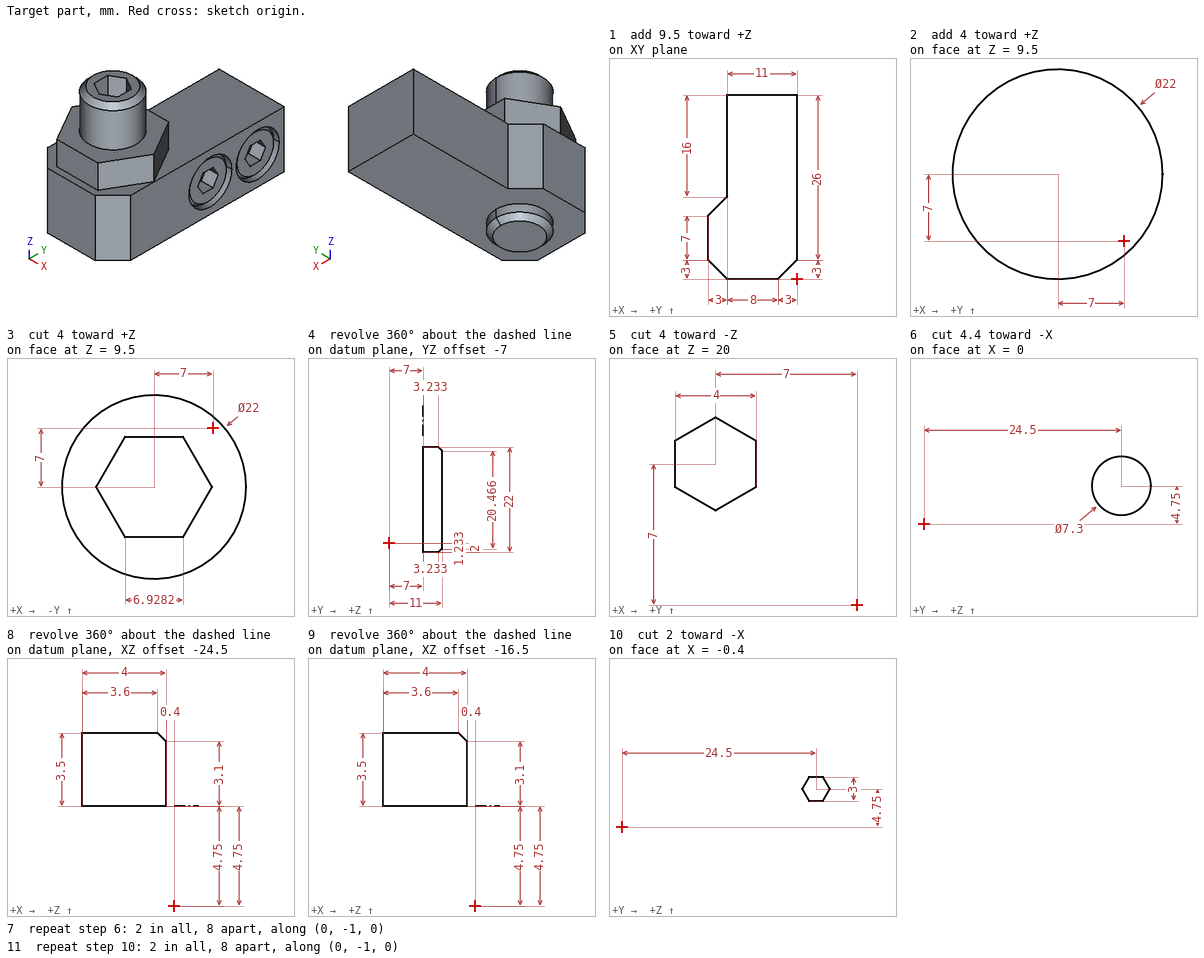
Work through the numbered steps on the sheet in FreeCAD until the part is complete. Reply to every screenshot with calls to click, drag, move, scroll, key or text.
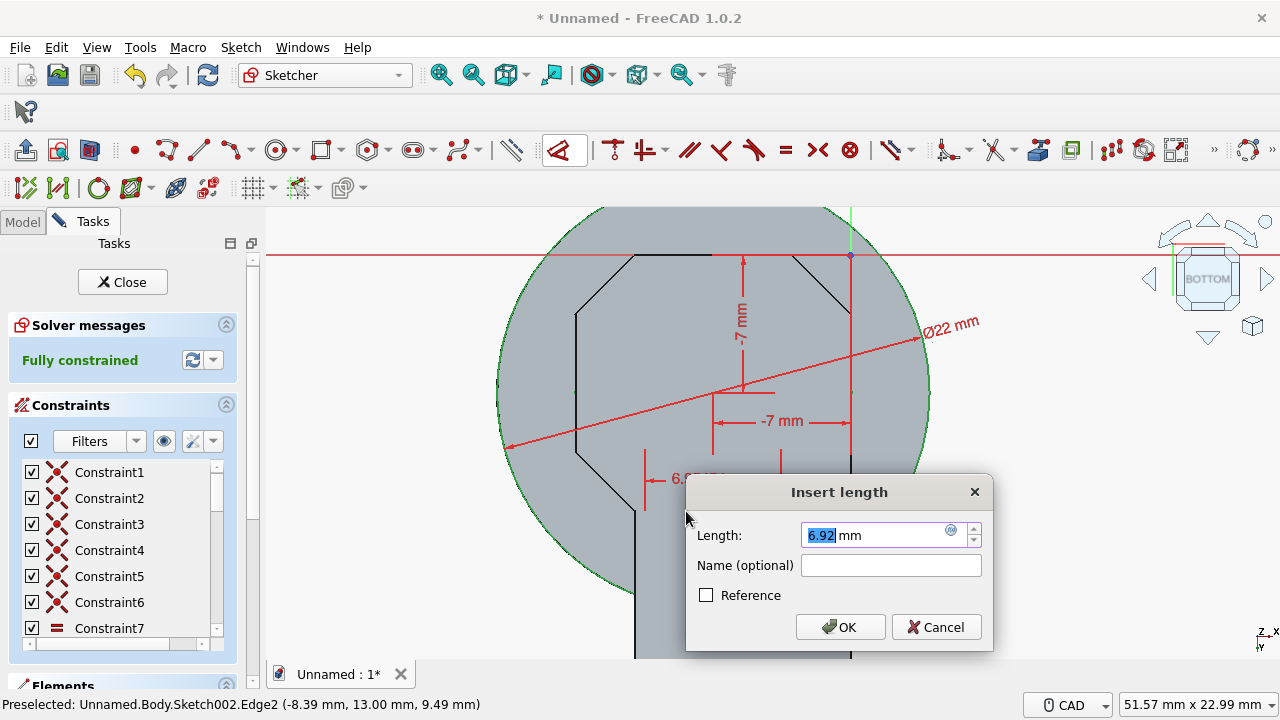
text(6.9282)
key(Return)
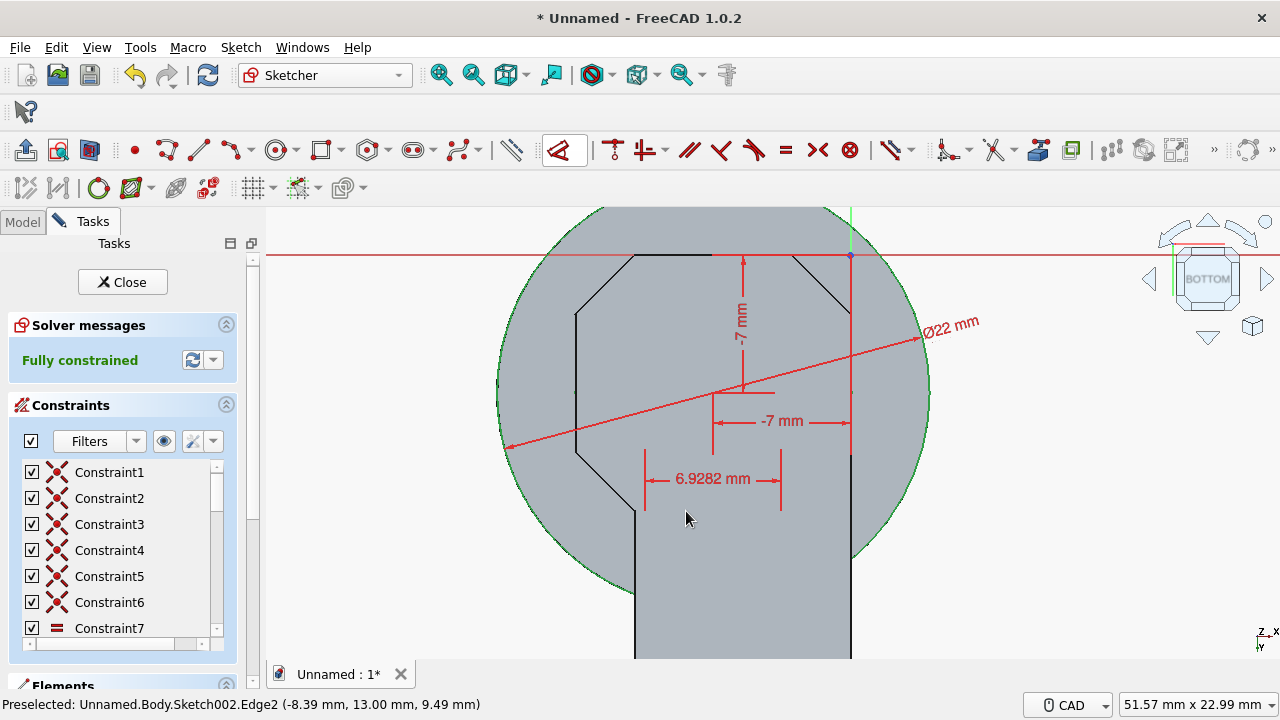
click(123, 282)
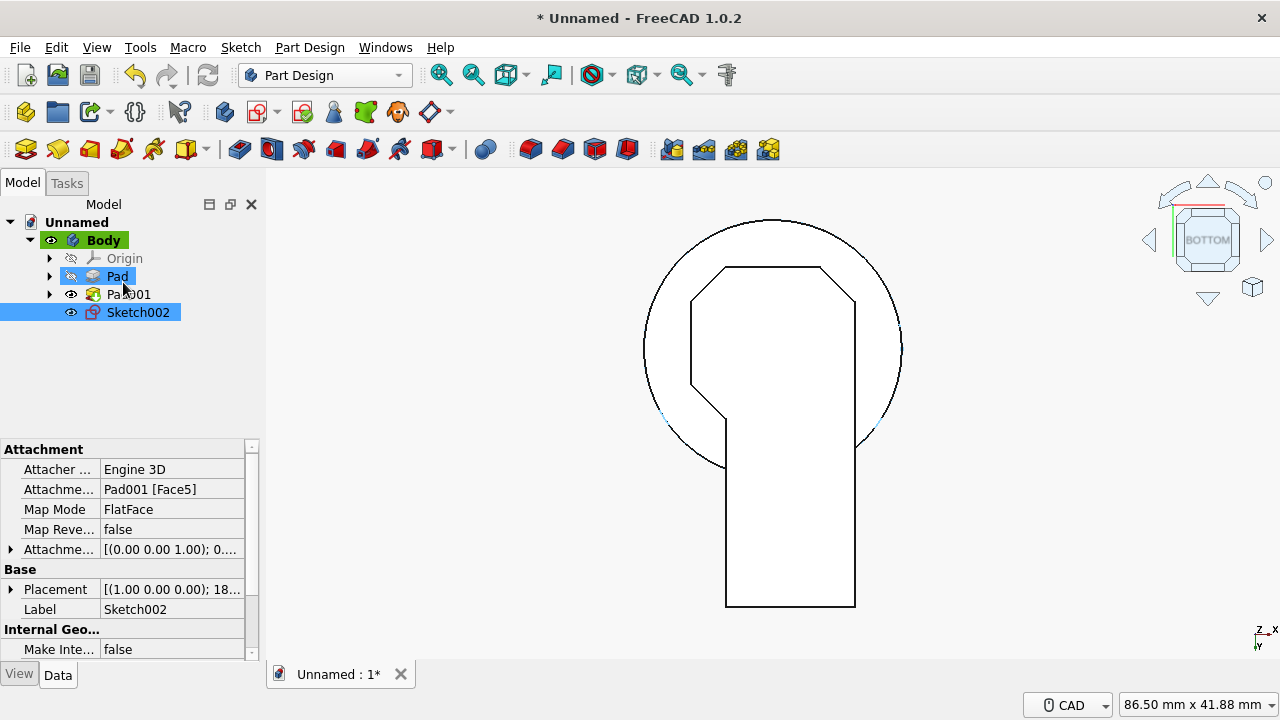
click(240, 150)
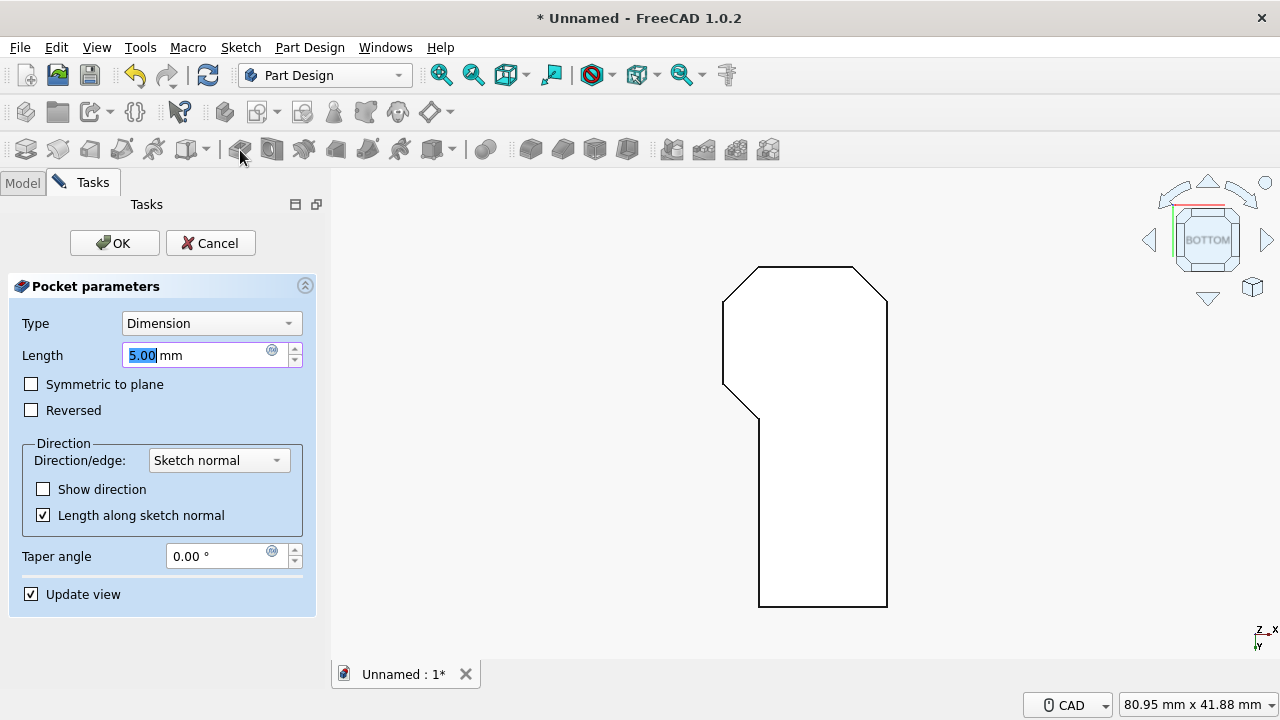
text(4)
key(Tab)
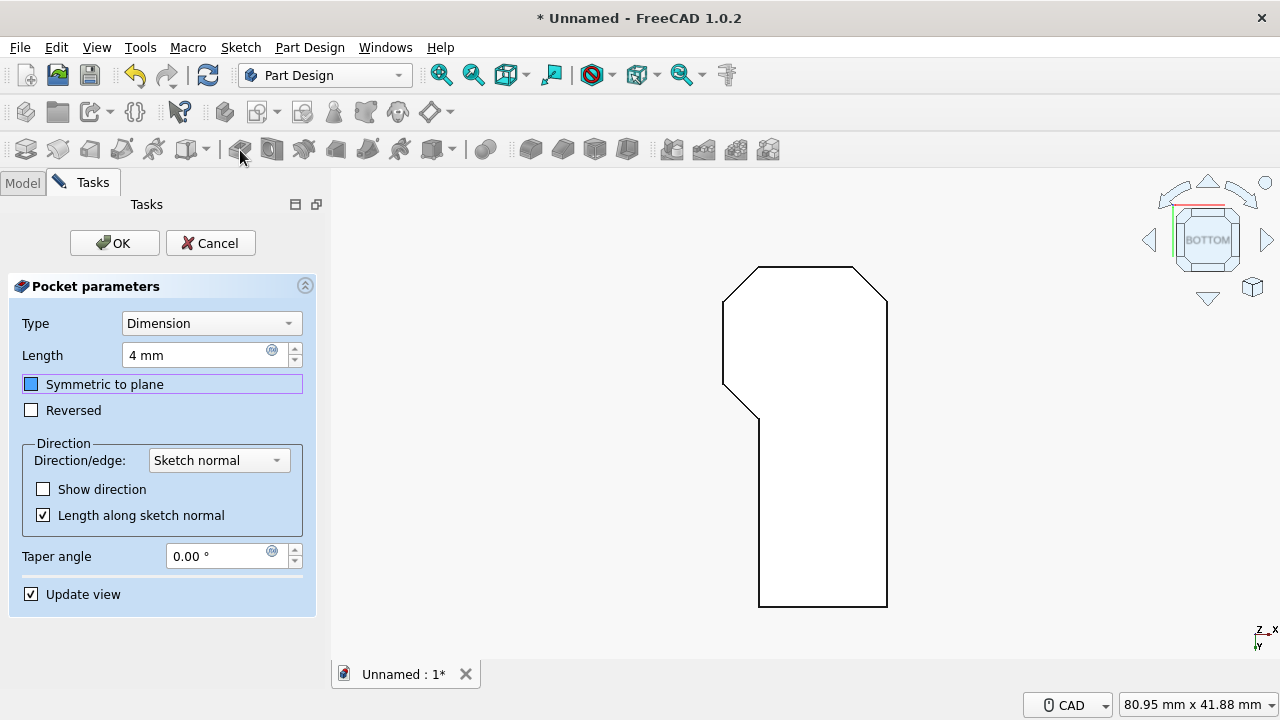
click(115, 243)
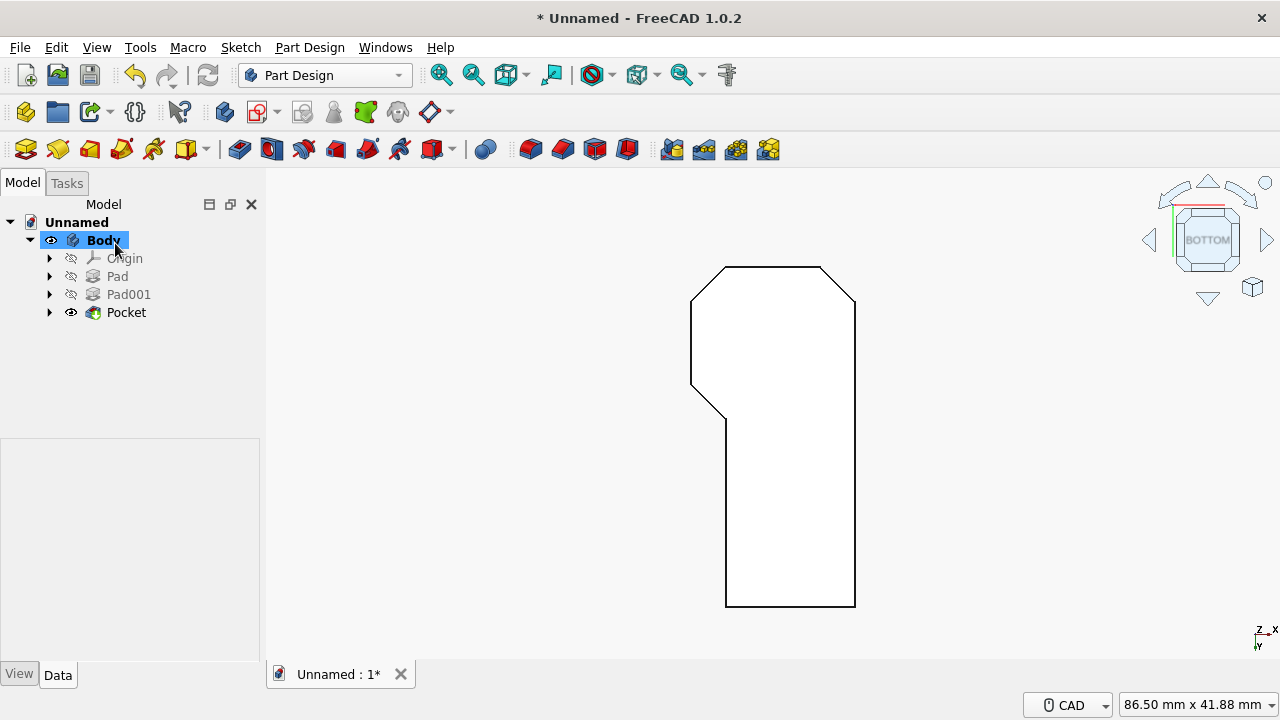
click(50, 258)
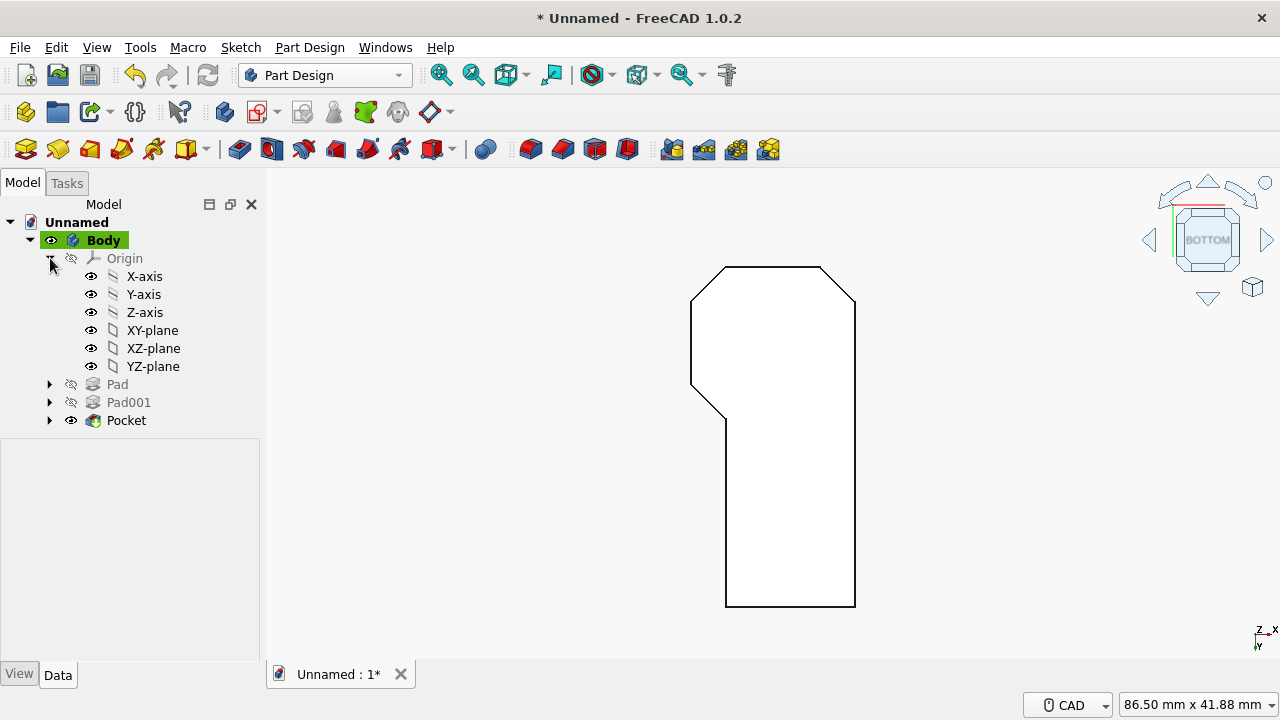
click(136, 366)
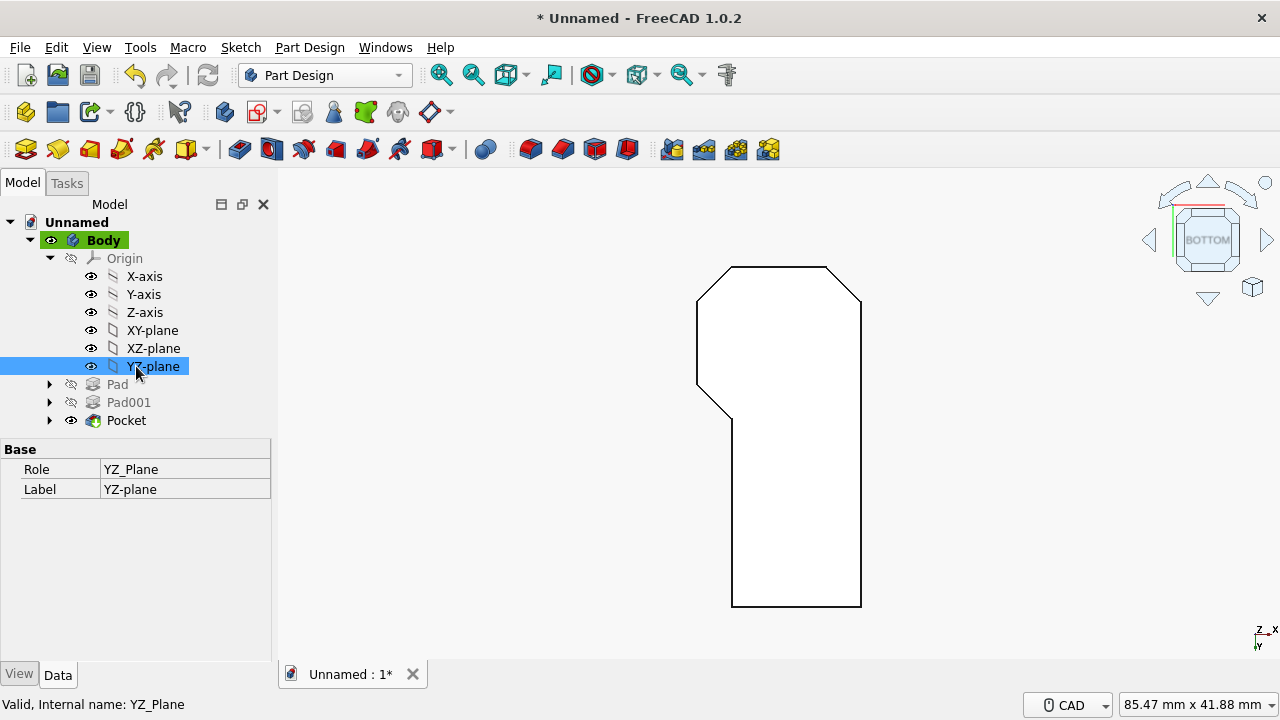
click(430, 112)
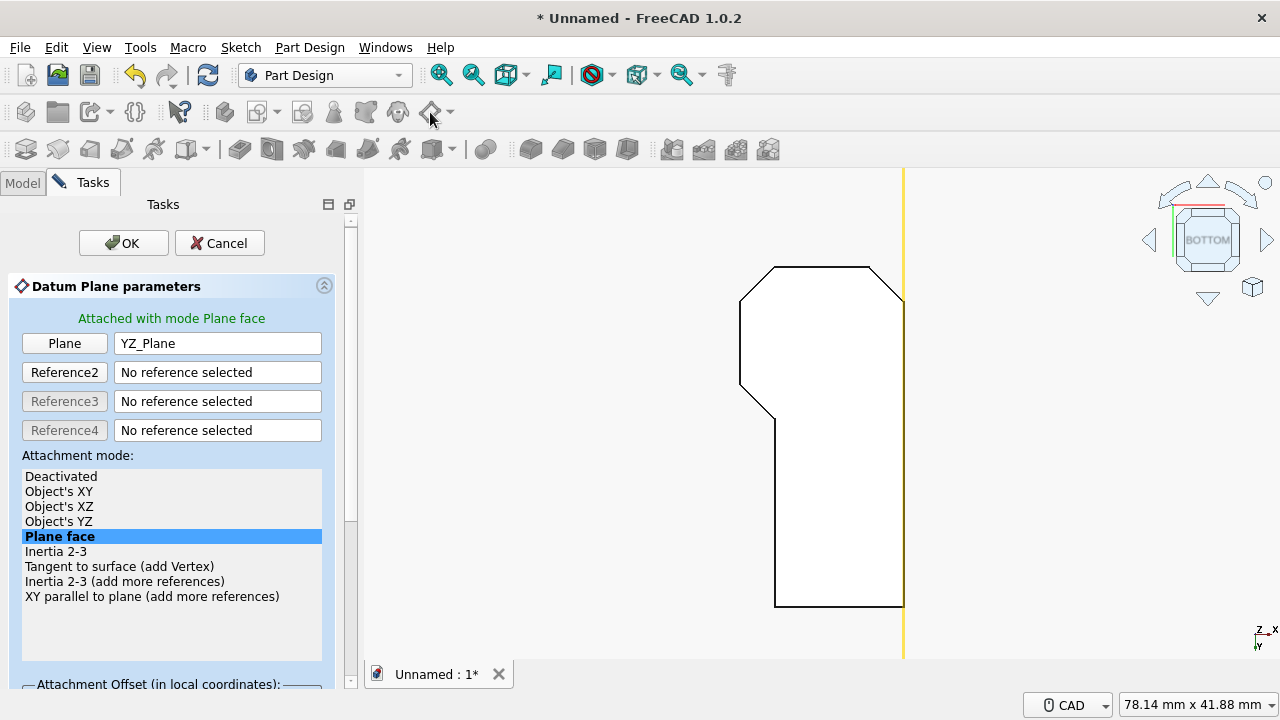
scroll(351, 451, down, 3)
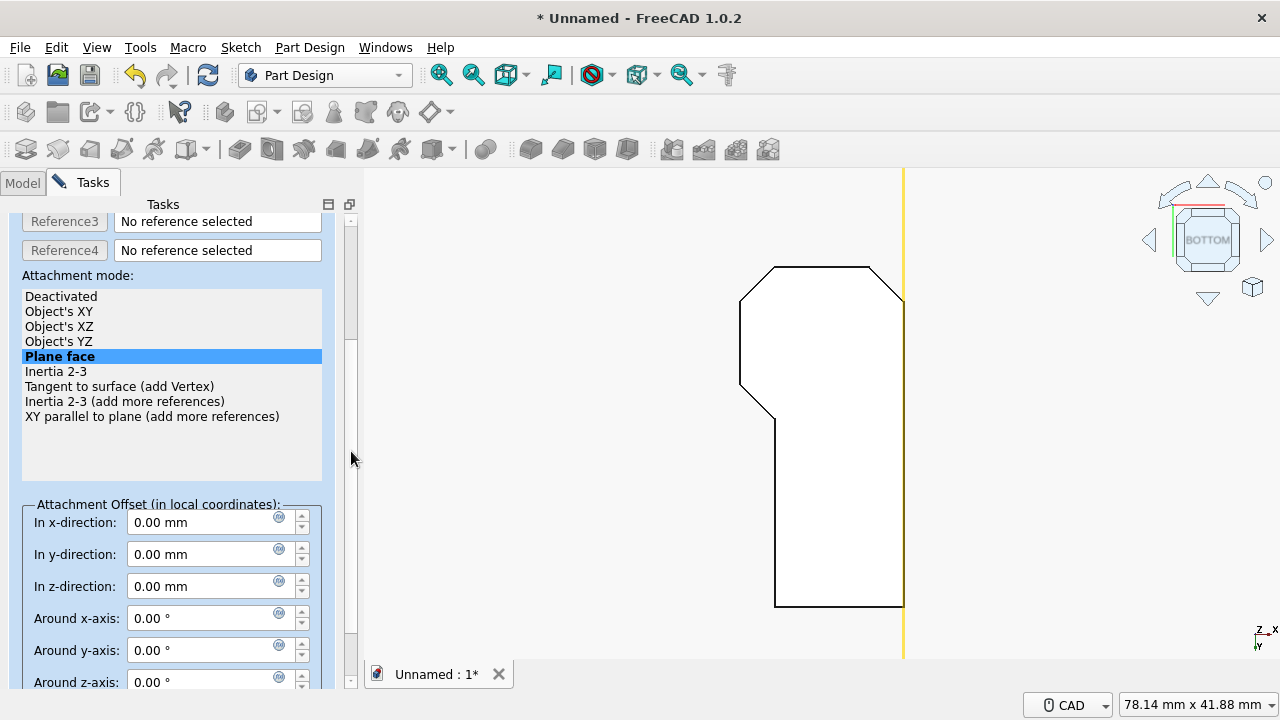
triple_click(210, 586)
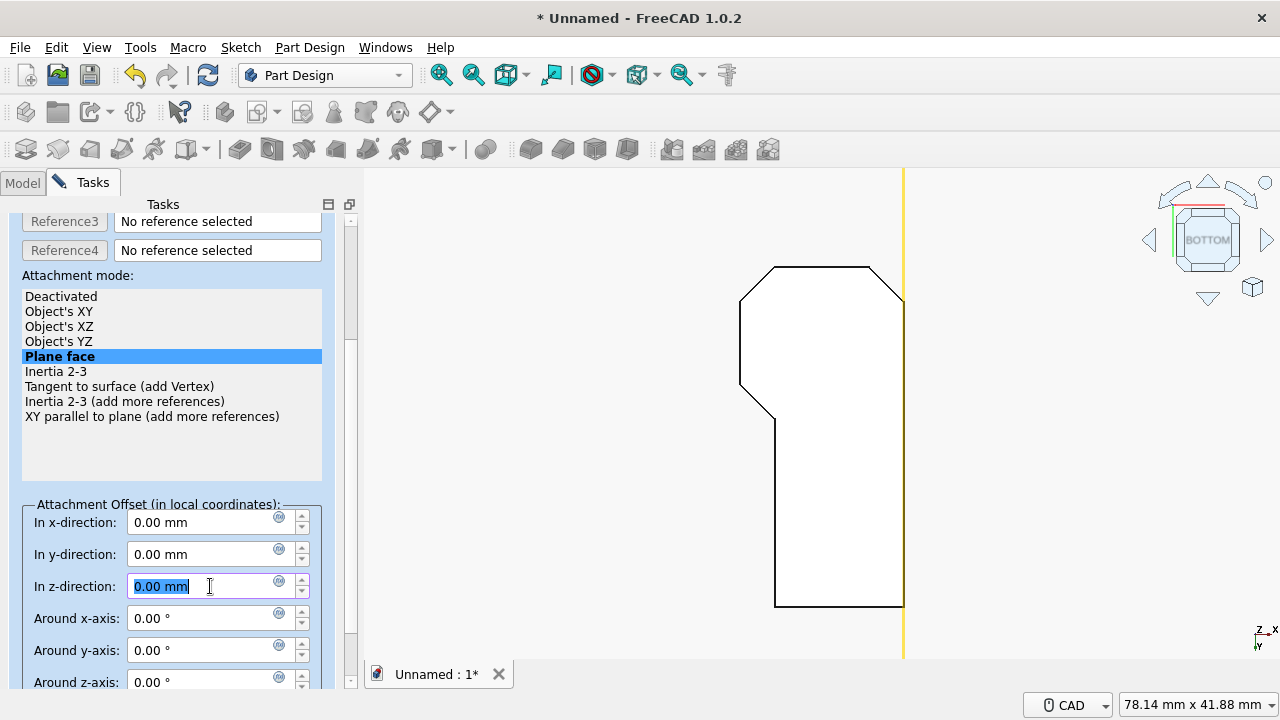
text(-7)
key(Tab)